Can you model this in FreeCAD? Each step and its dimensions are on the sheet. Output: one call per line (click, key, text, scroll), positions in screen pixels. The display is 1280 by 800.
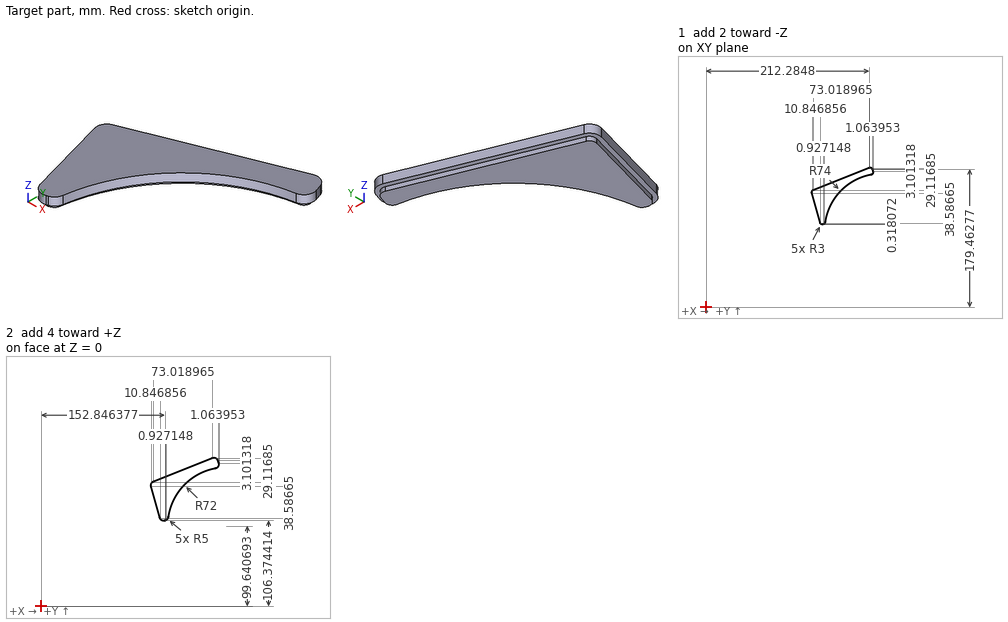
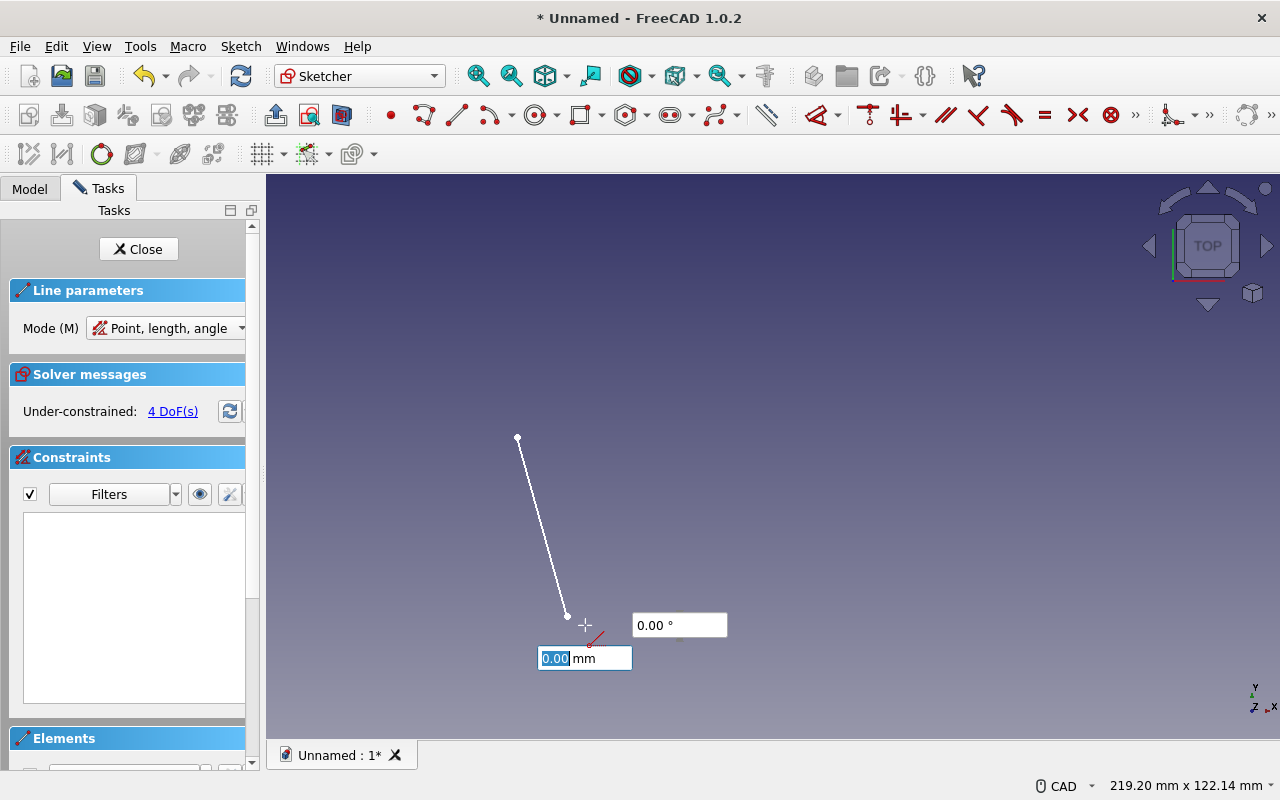
scroll(589, 623, up, 7)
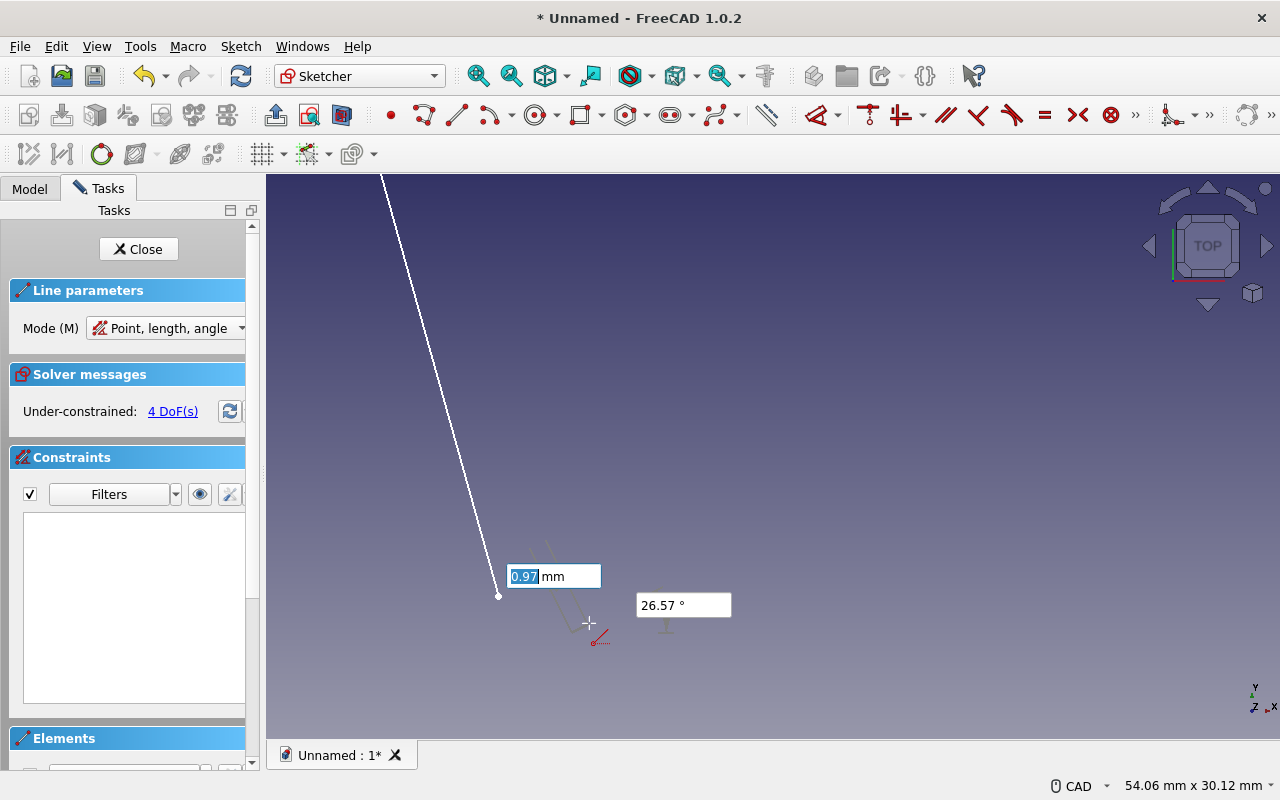
click(590, 622)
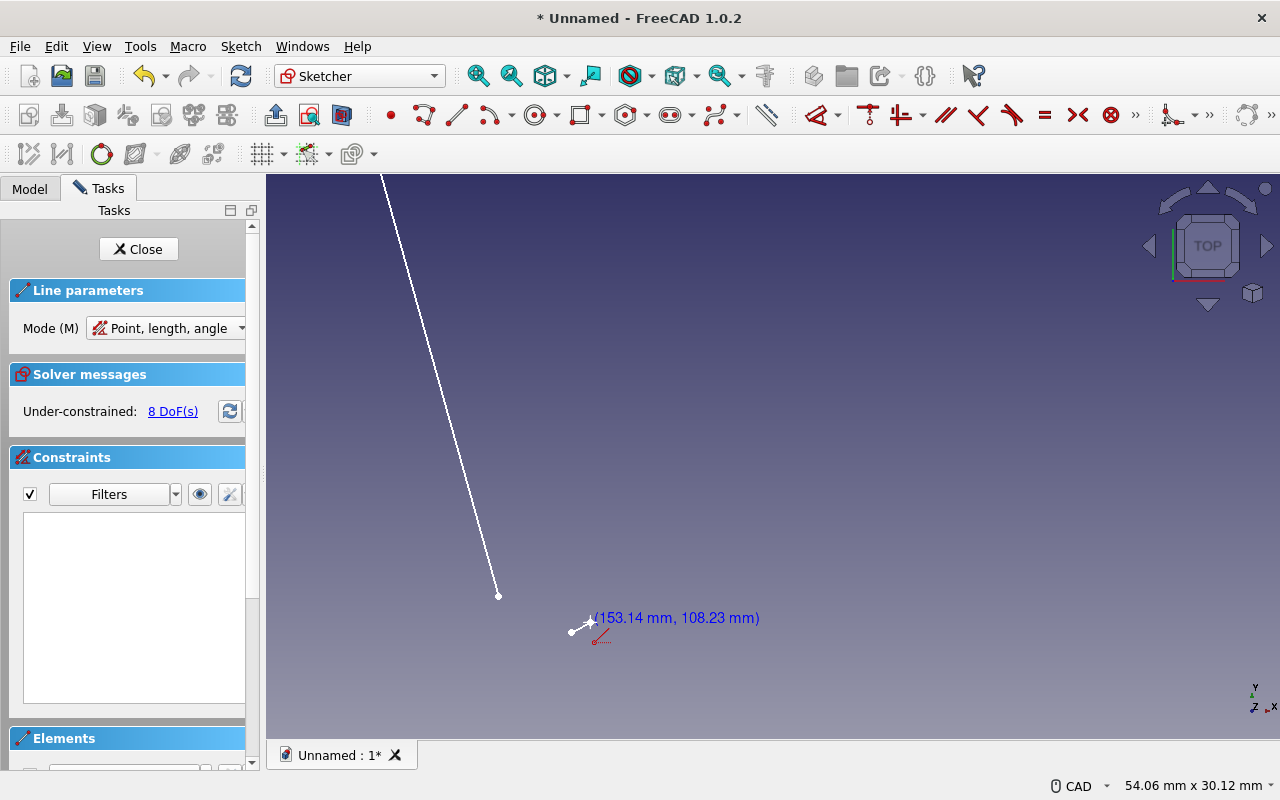
scroll(593, 625, down, 7)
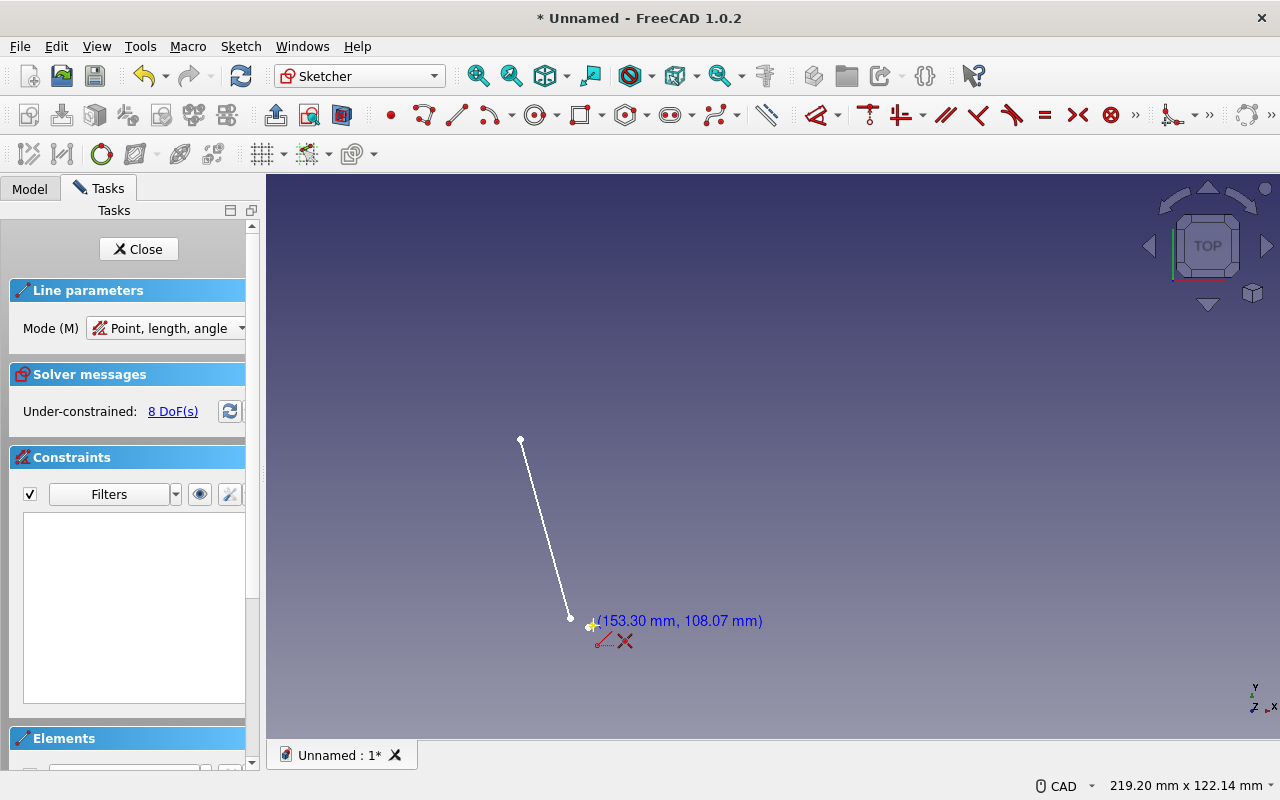
click(889, 310)
click(884, 296)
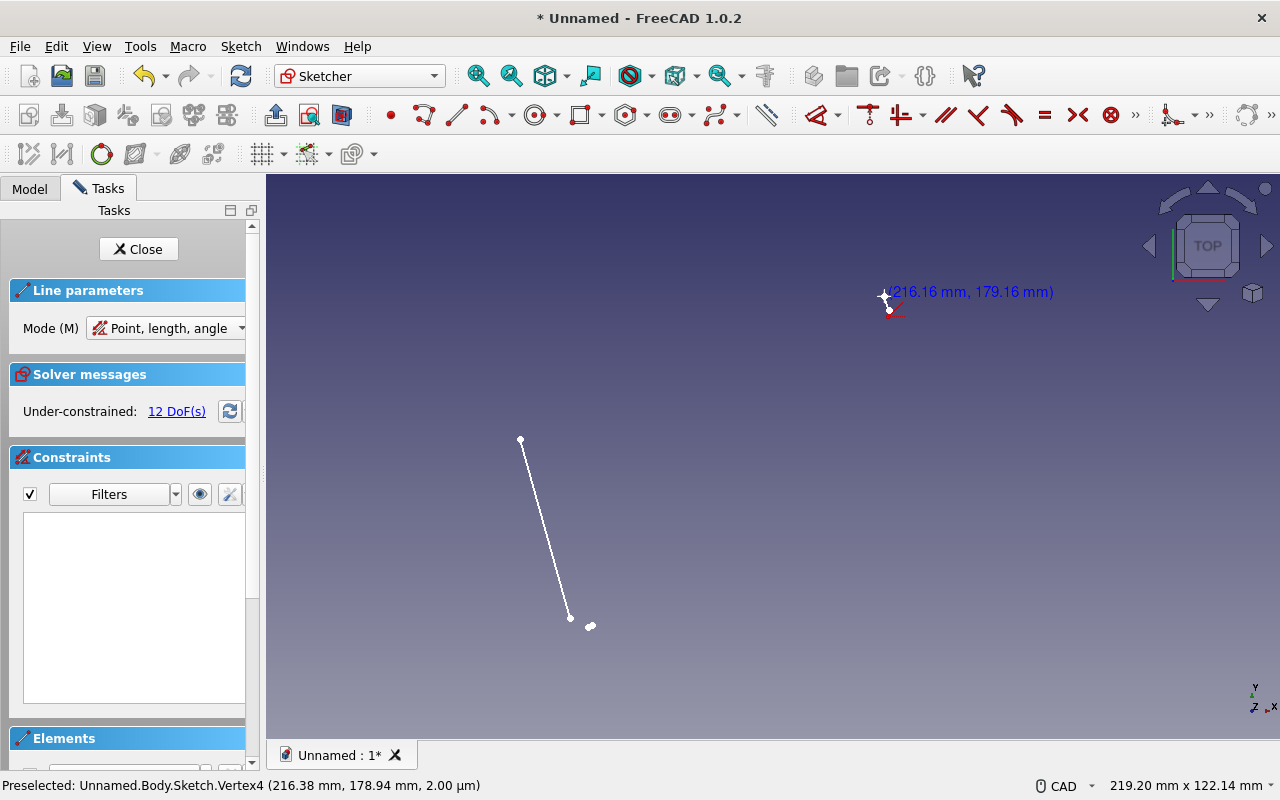
click(866, 287)
click(528, 422)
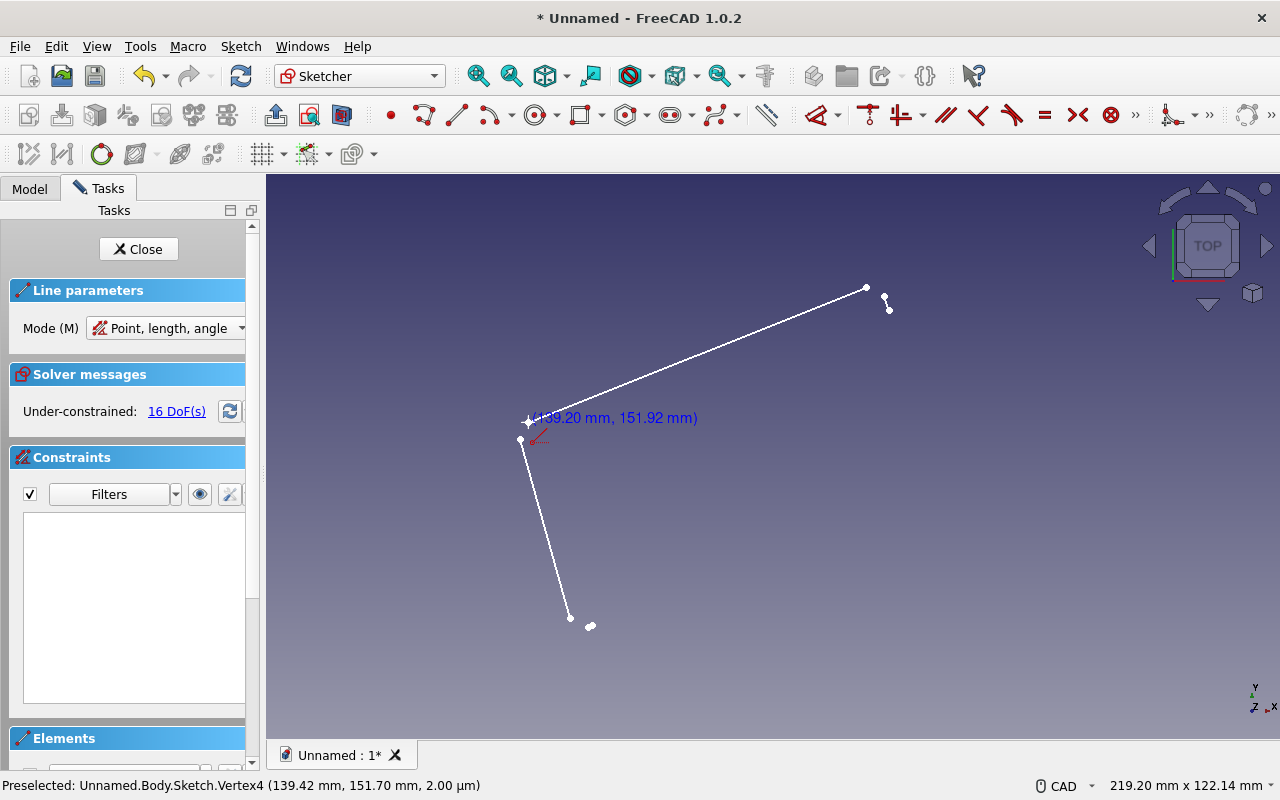
click(512, 116)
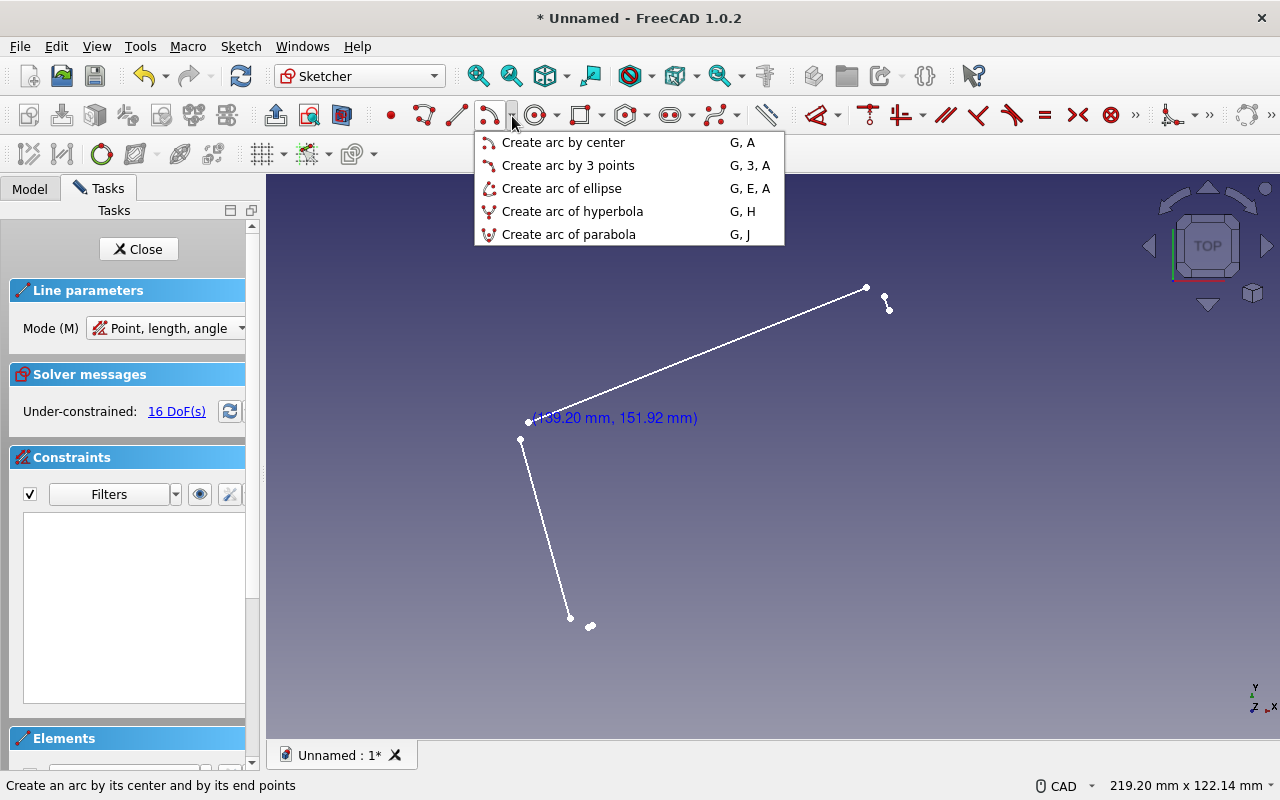
click(630, 166)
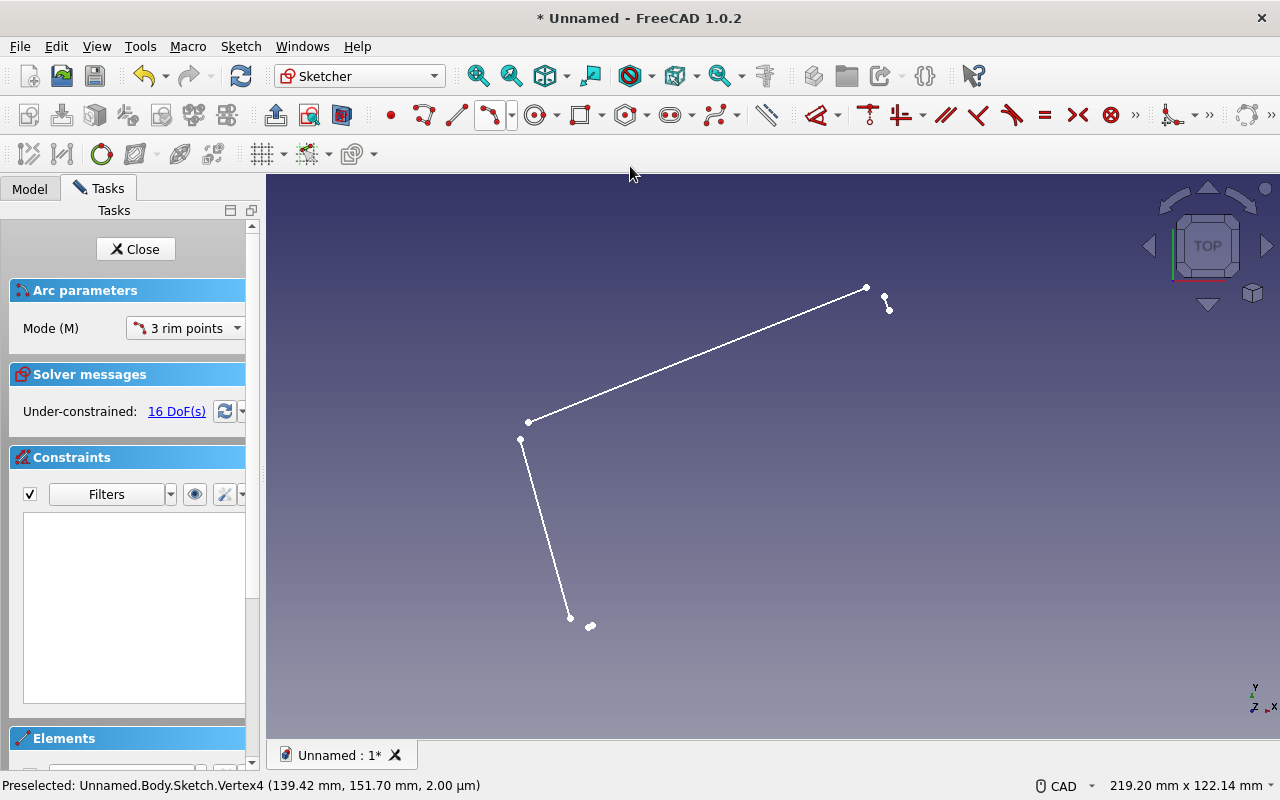
click(570, 619)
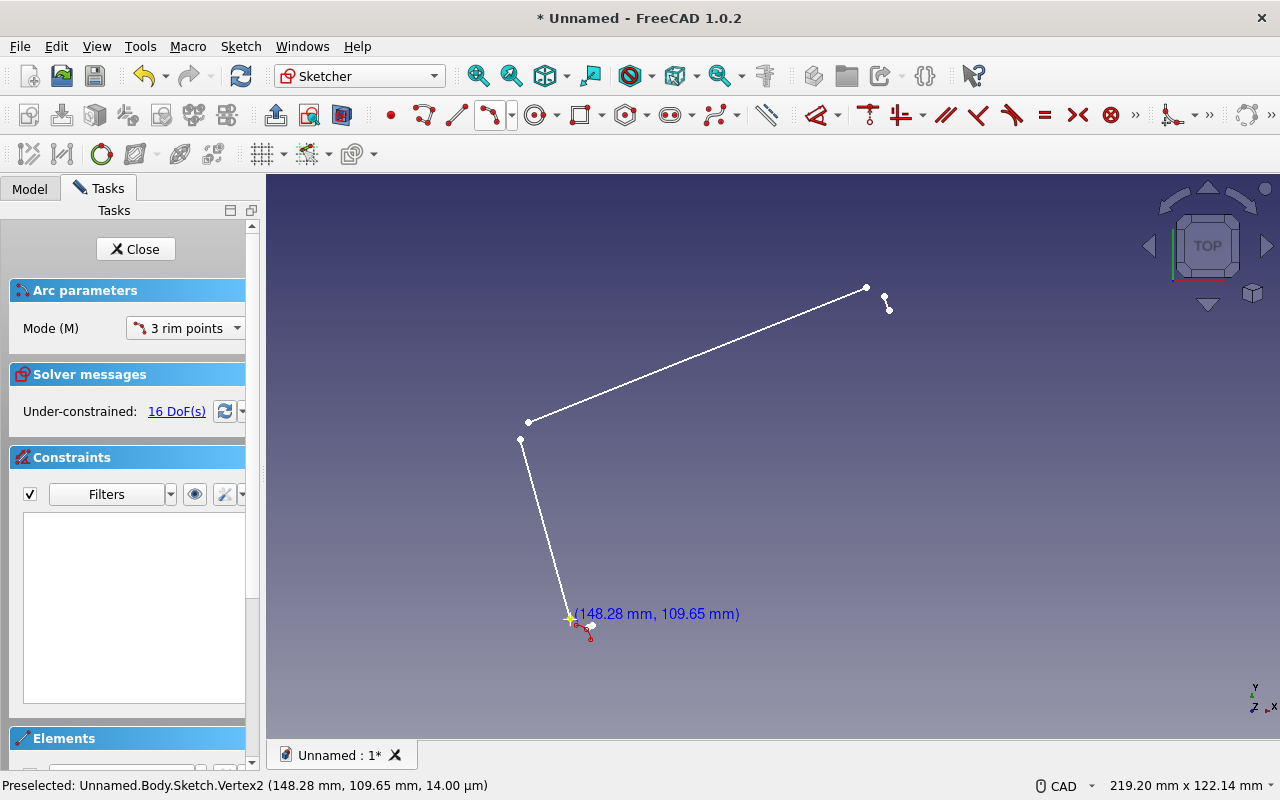
scroll(588, 626, up, 10)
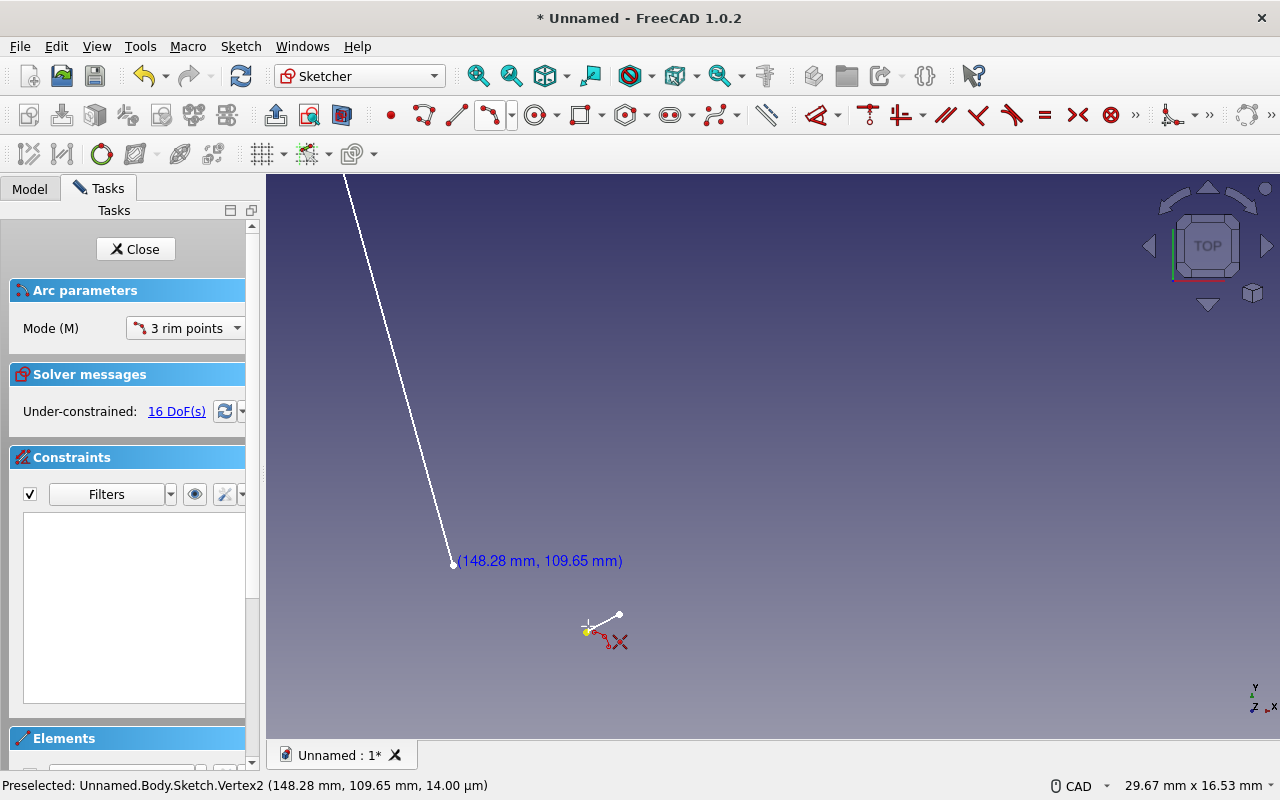
click(586, 632)
click(506, 618)